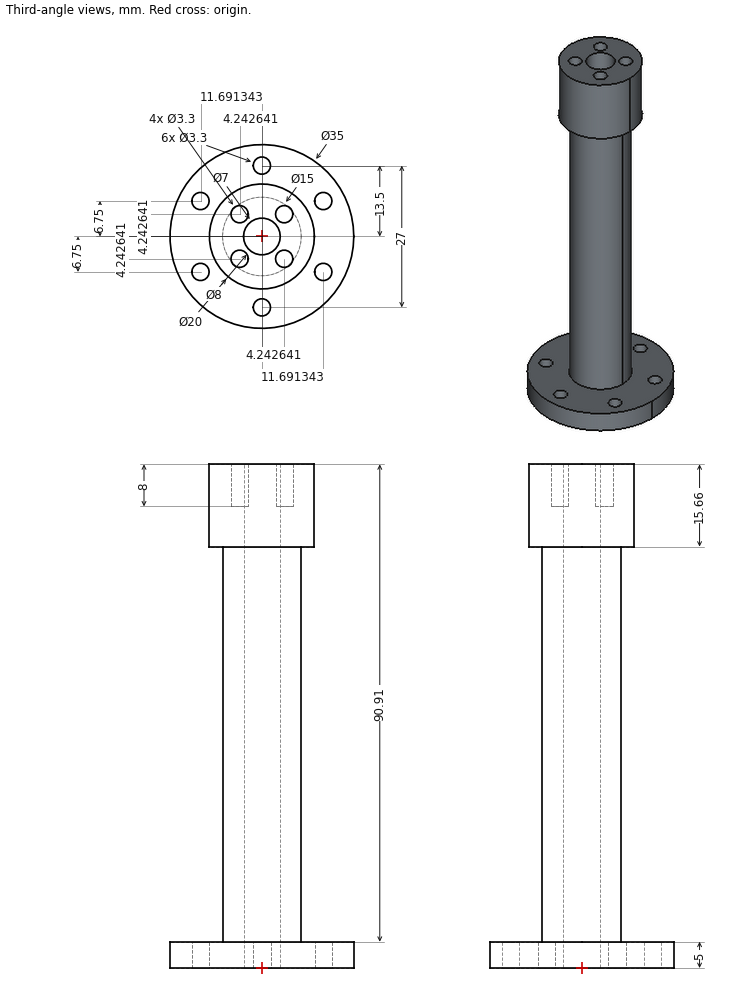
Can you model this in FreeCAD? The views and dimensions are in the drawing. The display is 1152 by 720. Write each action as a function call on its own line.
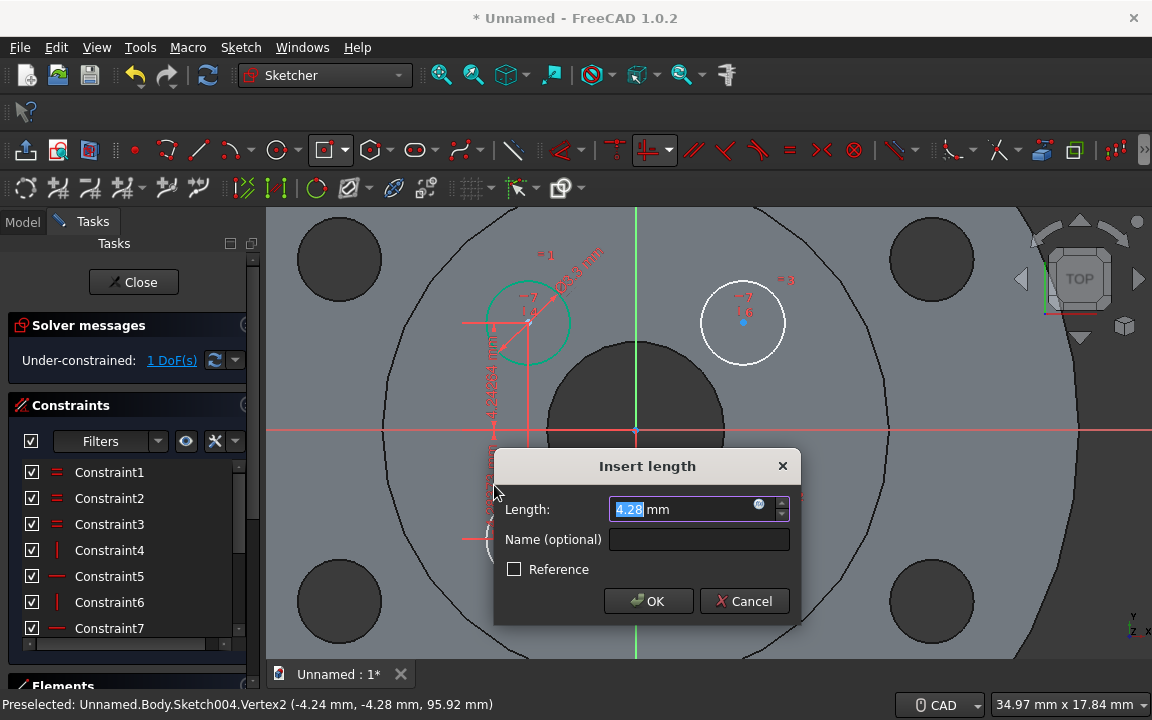
text(4.242641)
key(Return)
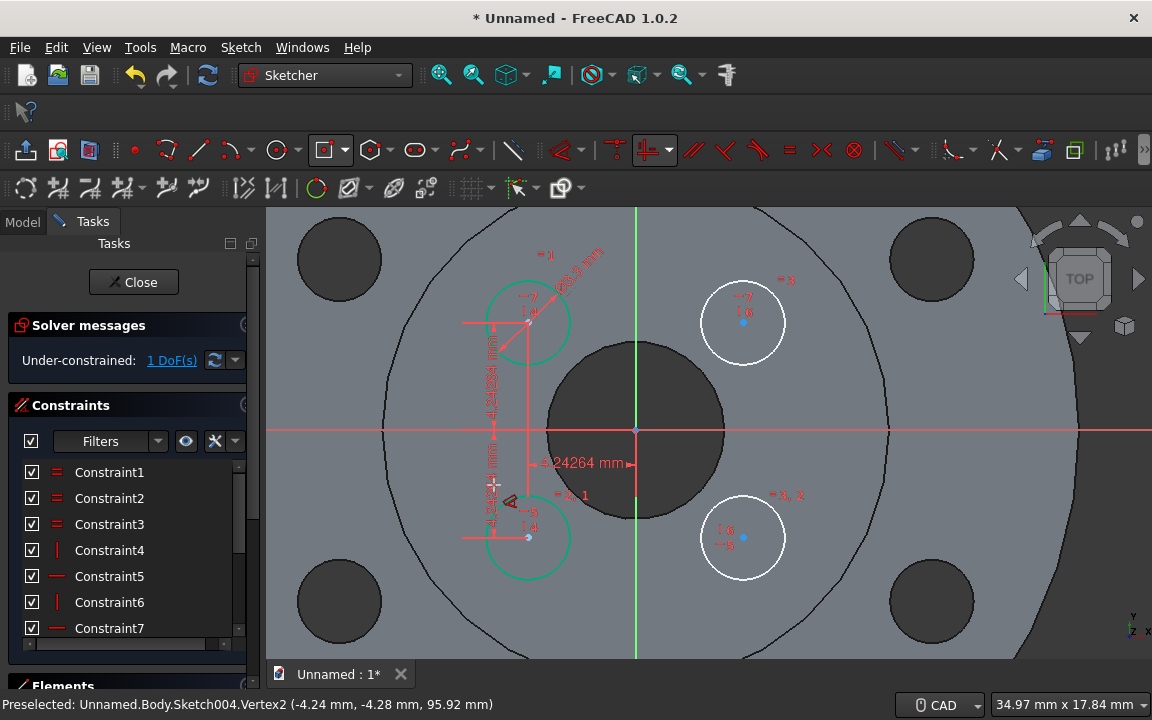
click(743, 538)
click(689, 572)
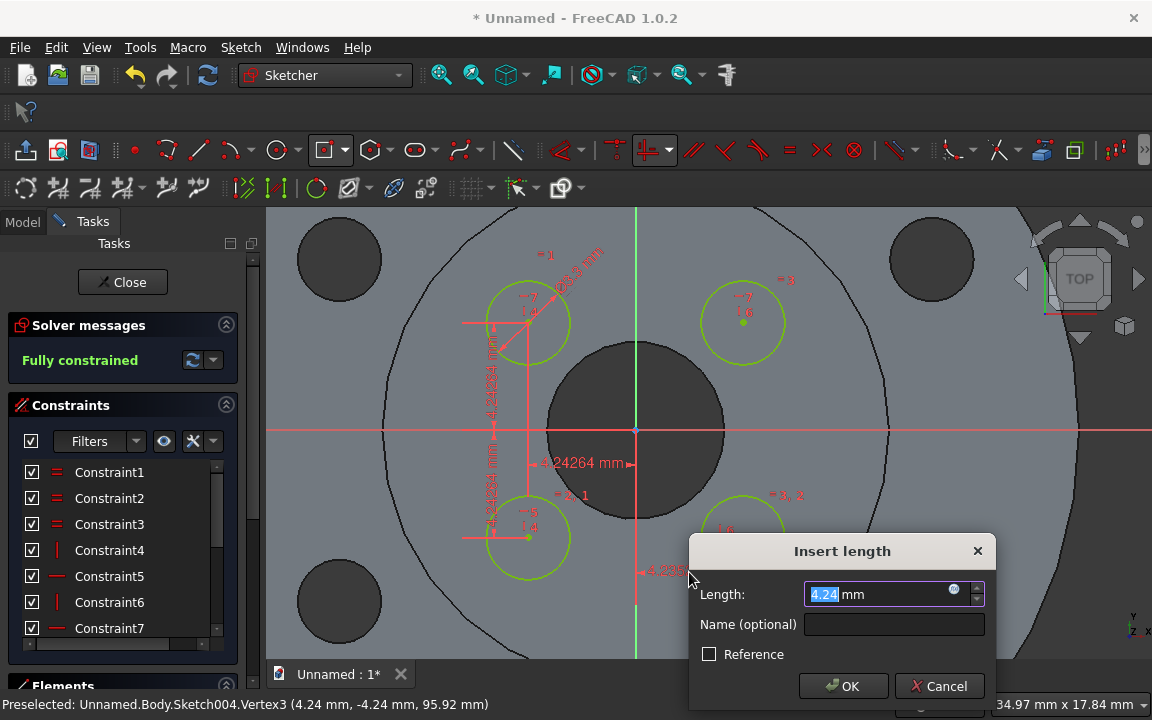
text(4.242641)
key(Return)
key(Escape)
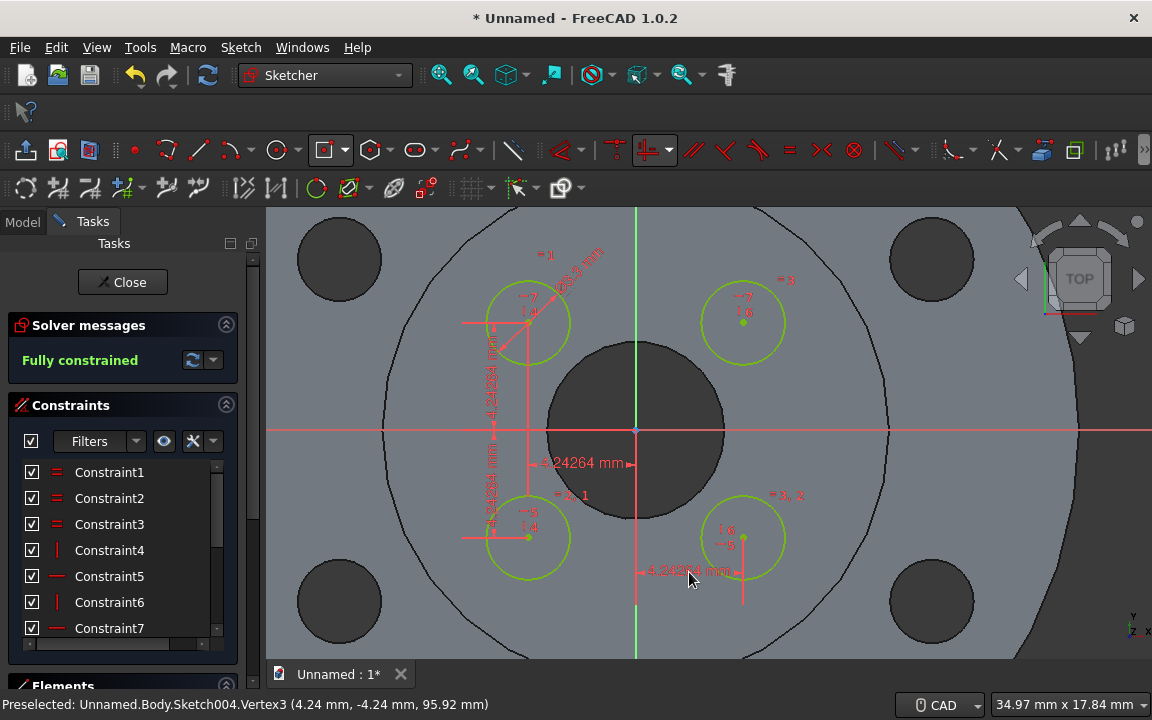
click(123, 282)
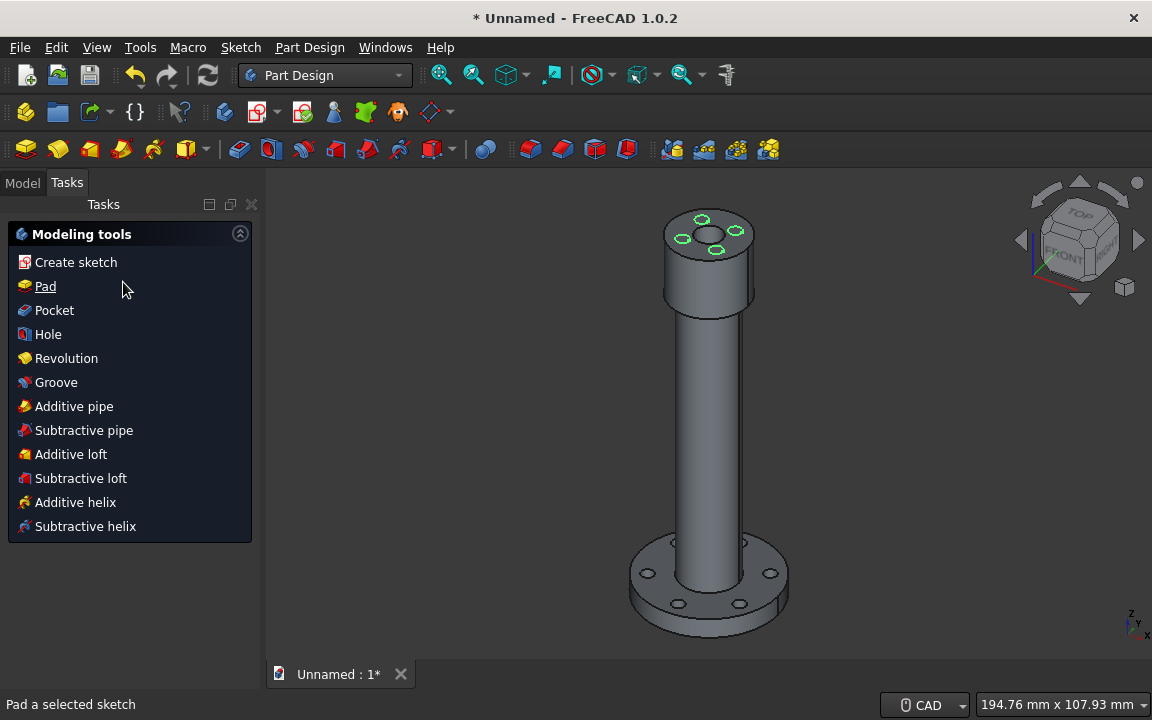
click(240, 150)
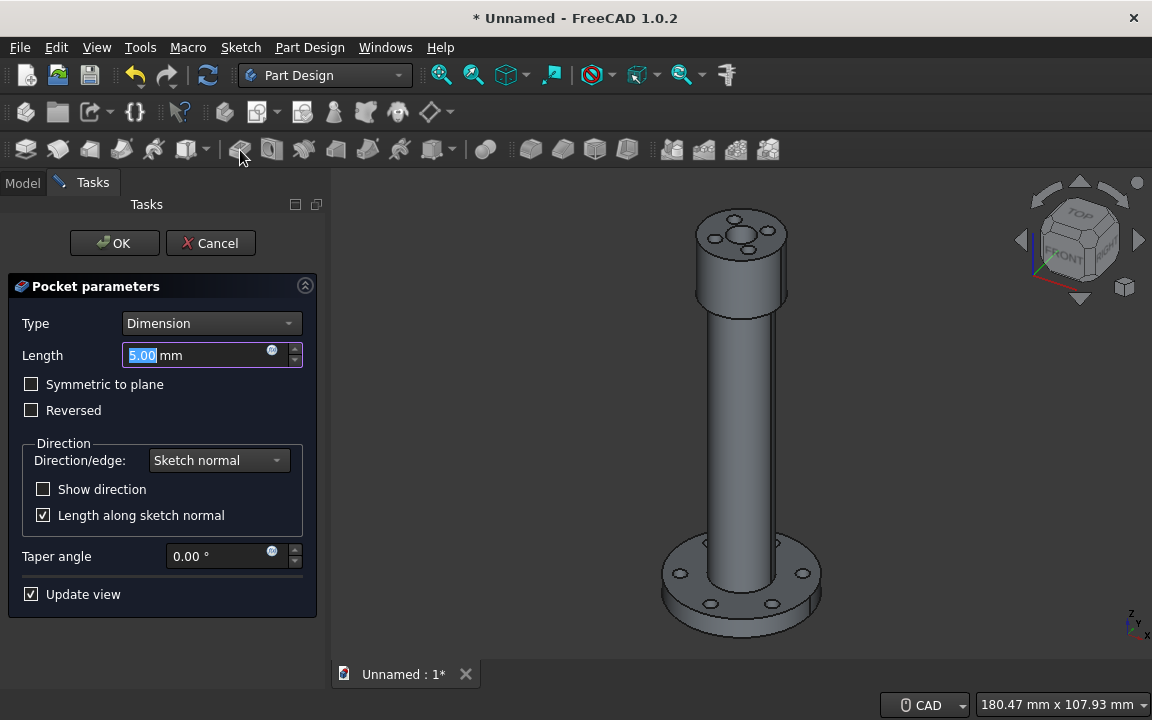
text(8)
key(Tab)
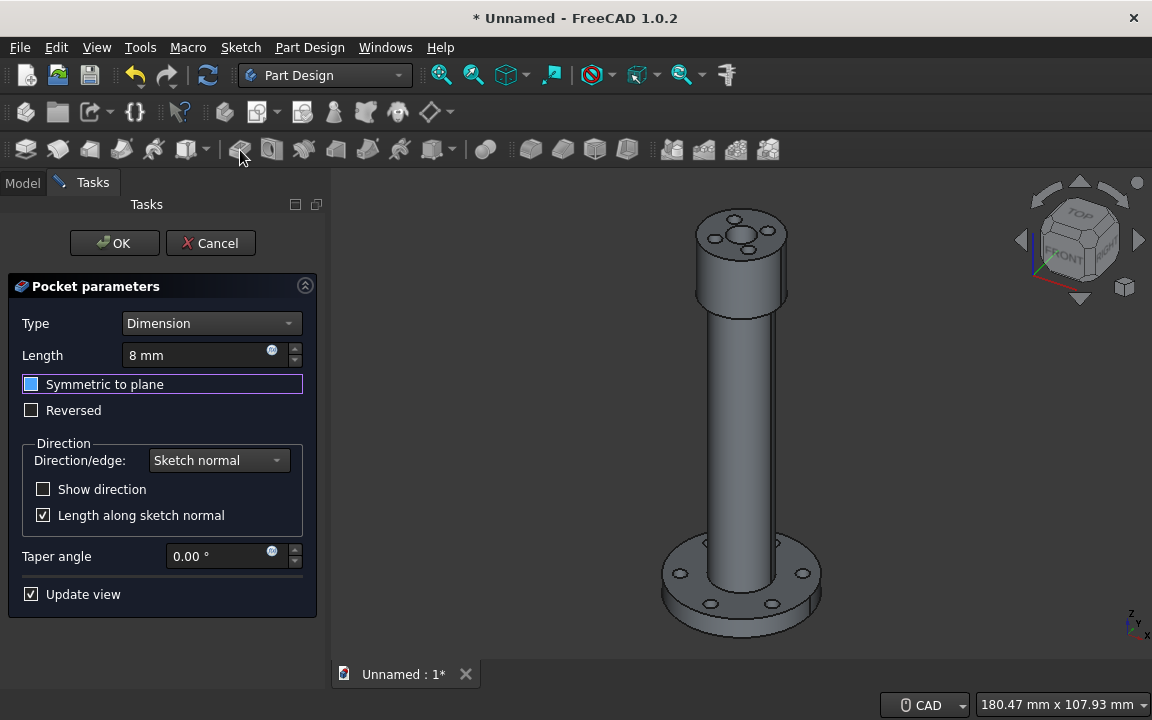
click(115, 243)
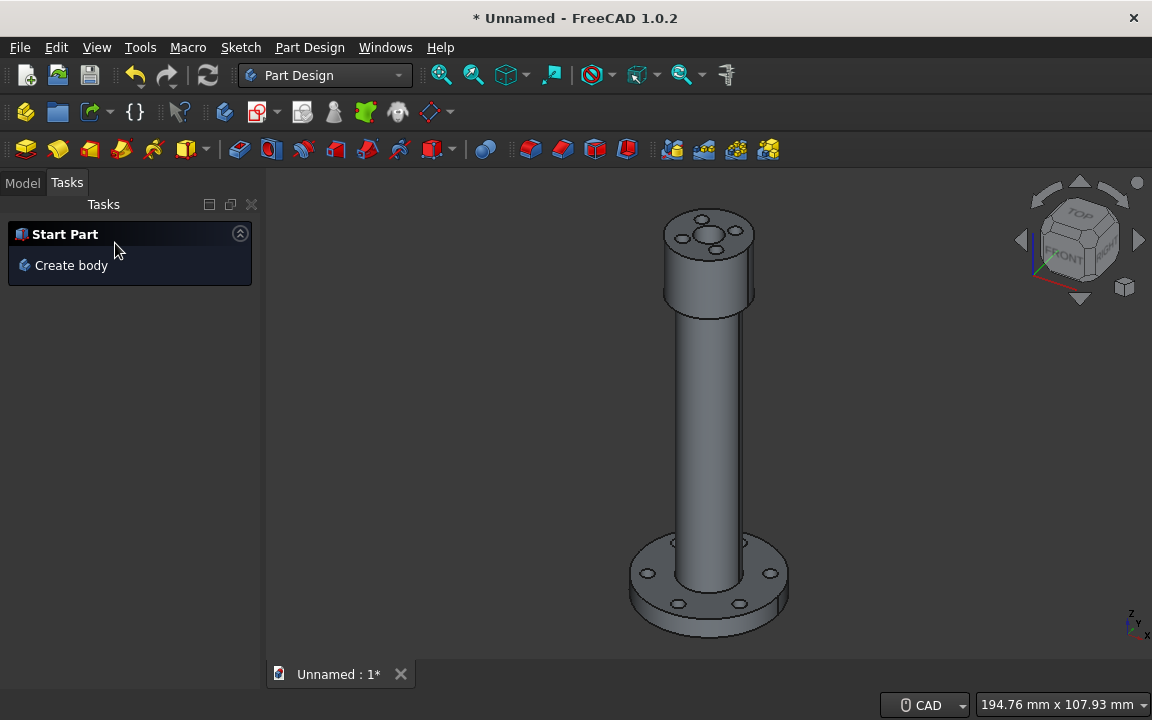
key(0)